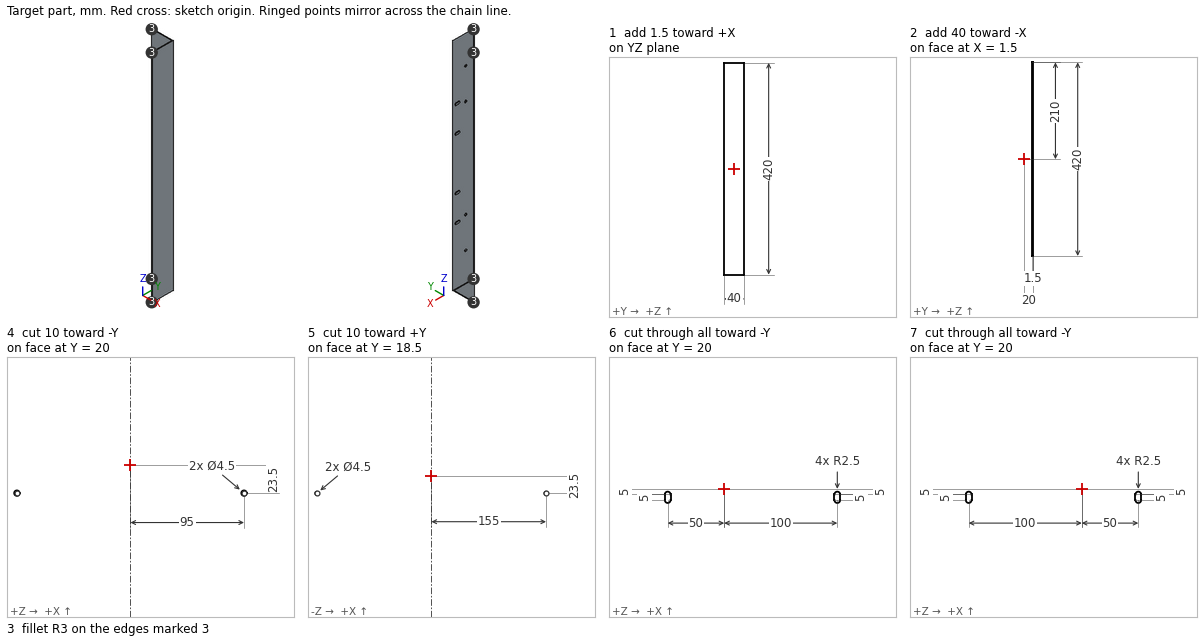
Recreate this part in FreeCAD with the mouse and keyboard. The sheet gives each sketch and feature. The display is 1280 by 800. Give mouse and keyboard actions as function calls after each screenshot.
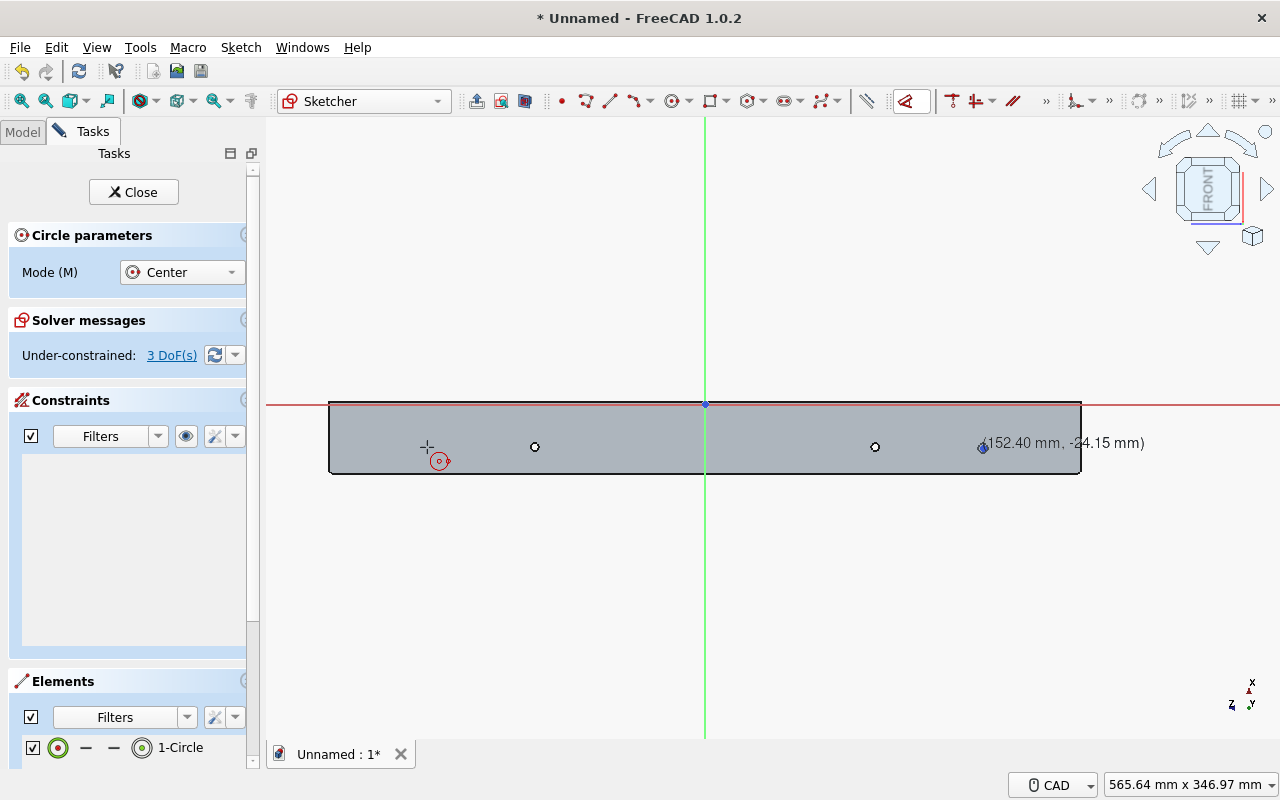
click(427, 447)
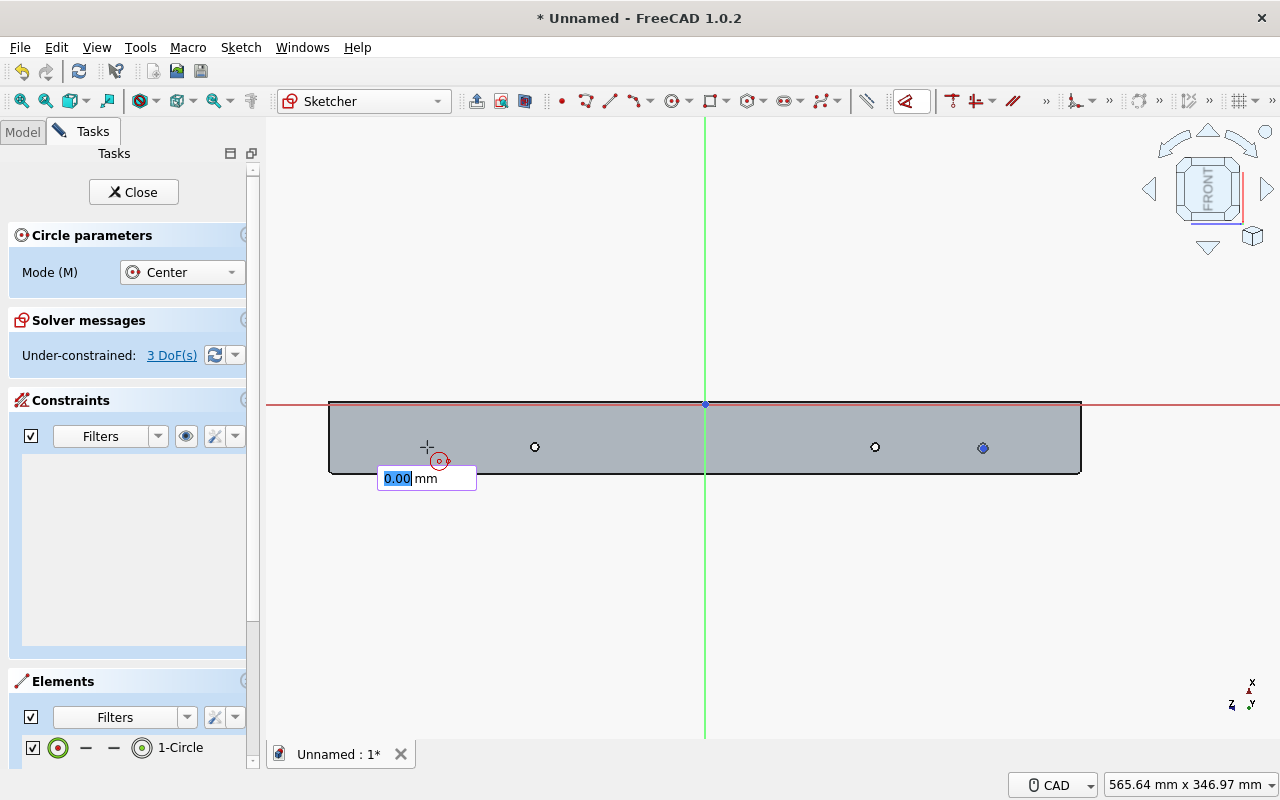
scroll(430, 444, up, 7)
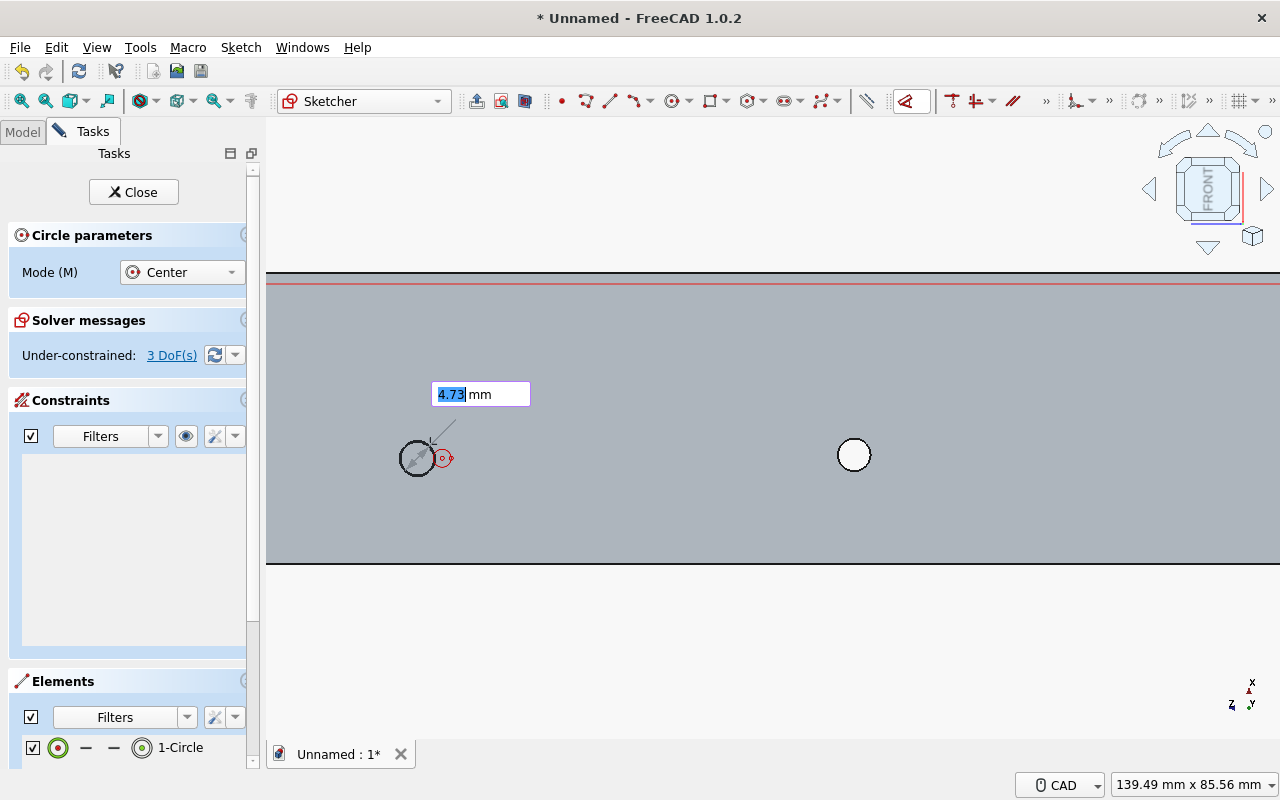
click(430, 443)
key(Escape)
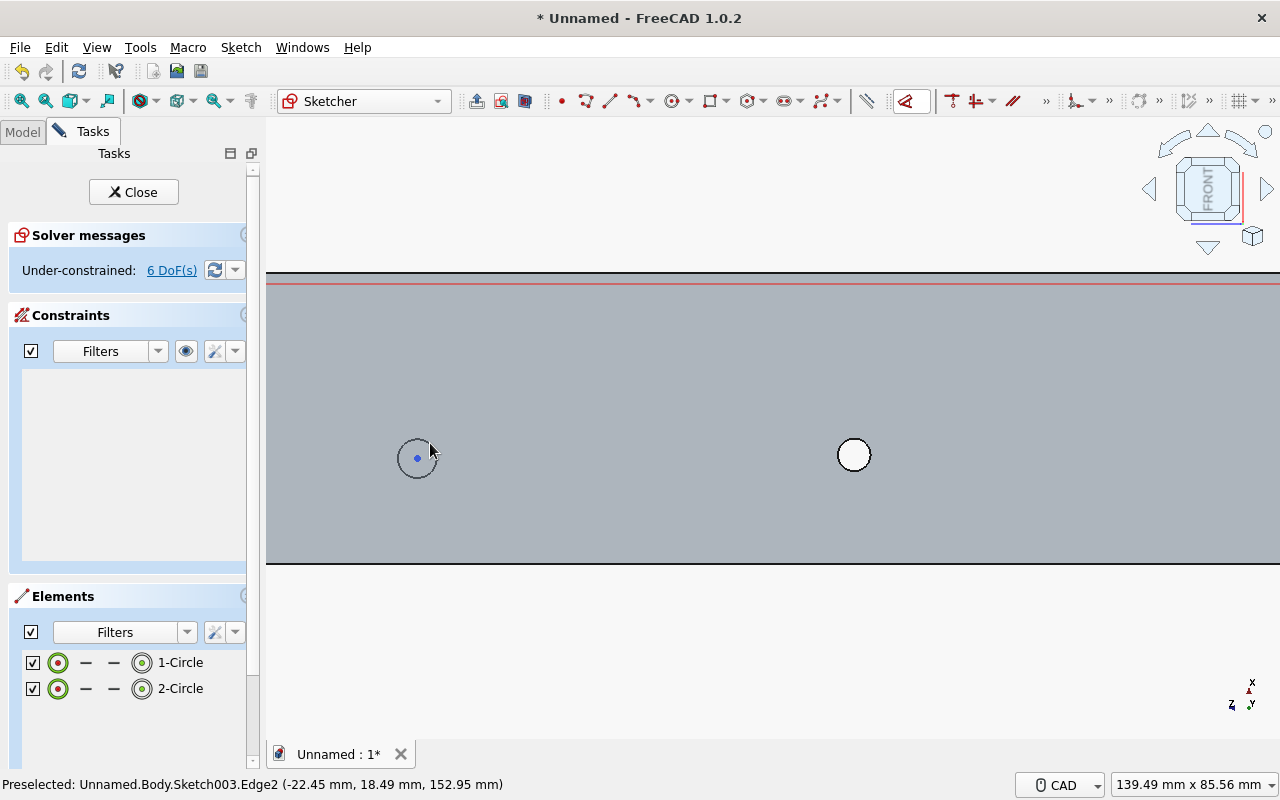
scroll(429, 444, down, 7)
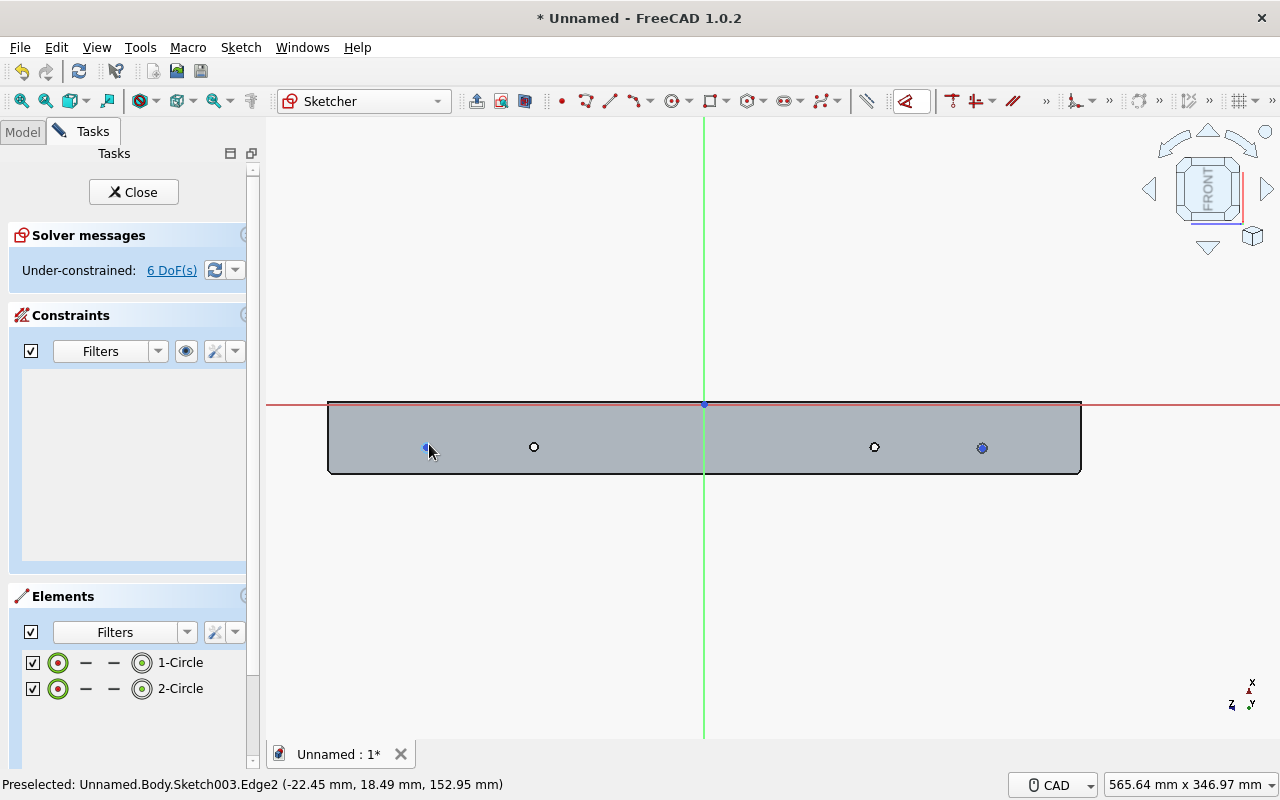
scroll(986, 445, up, 6)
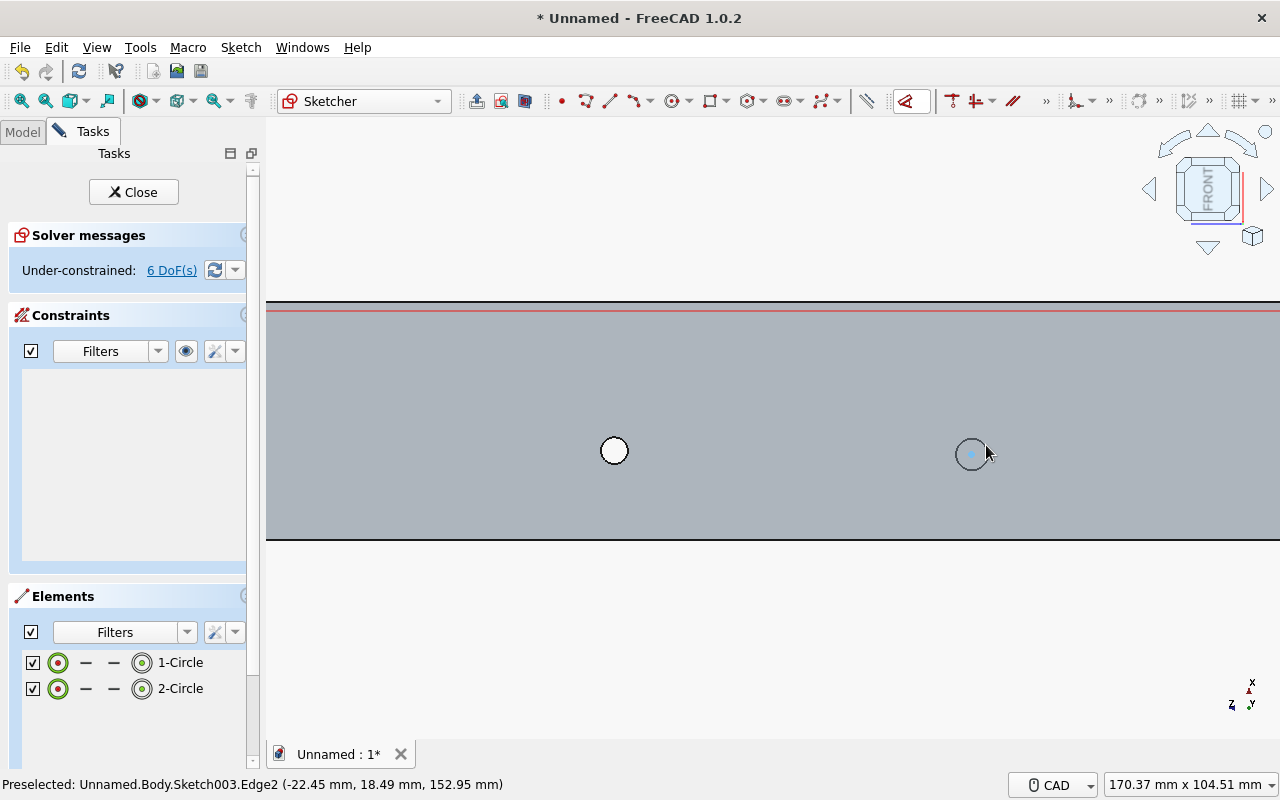
click(983, 443)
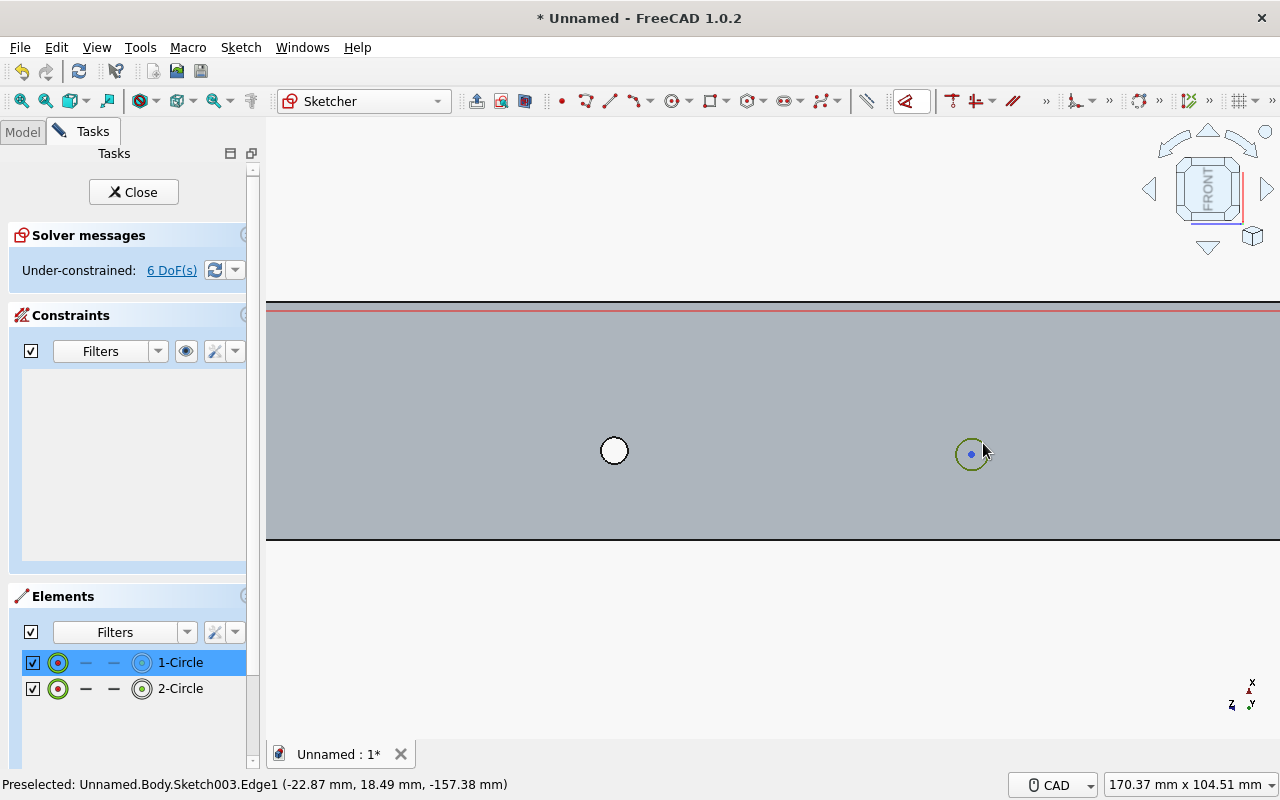
scroll(987, 445, down, 6)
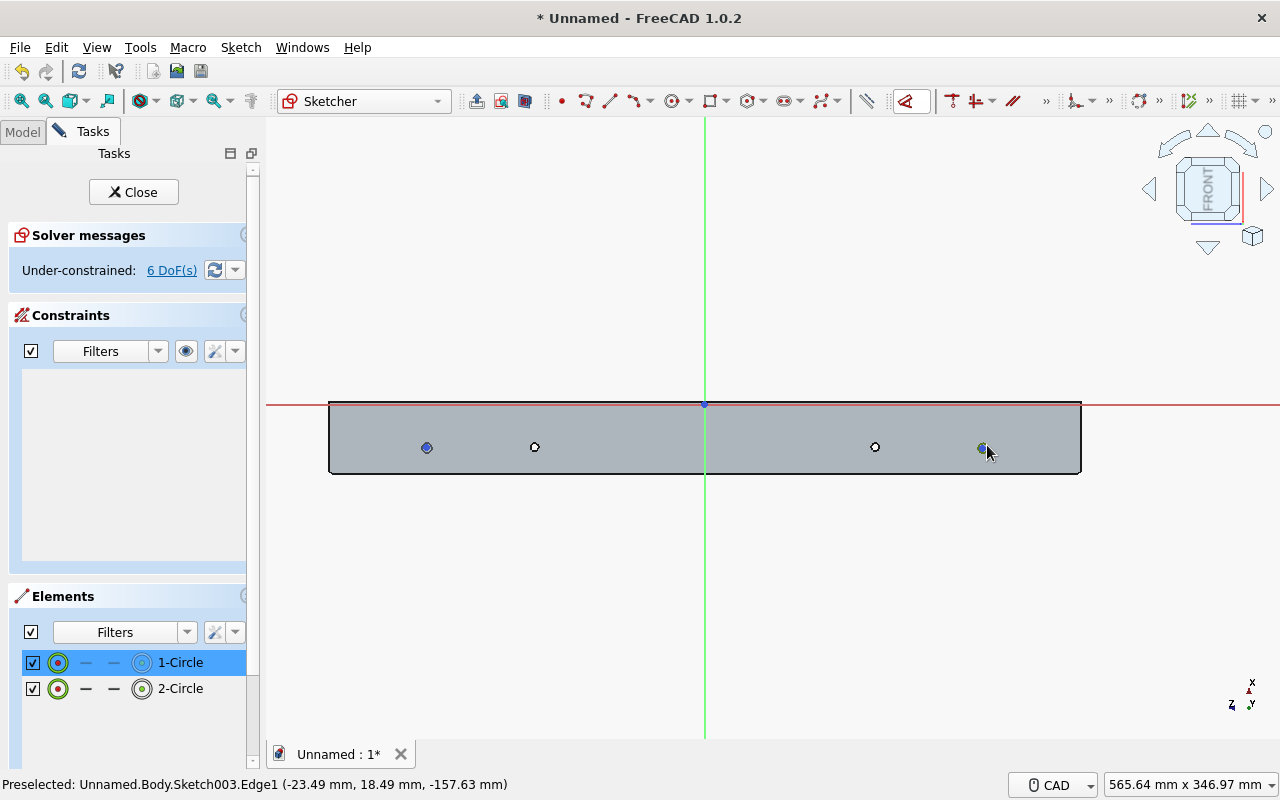
scroll(430, 445, up, 6)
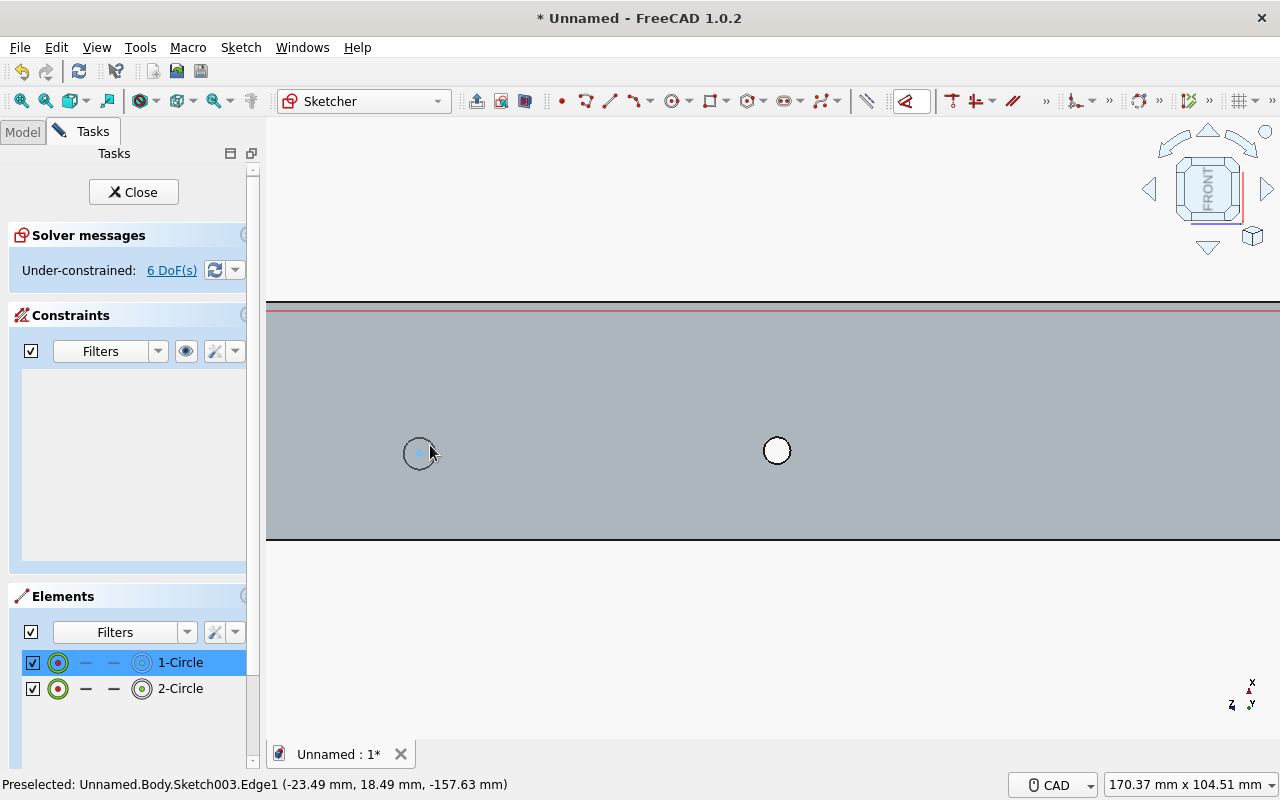
click(431, 443)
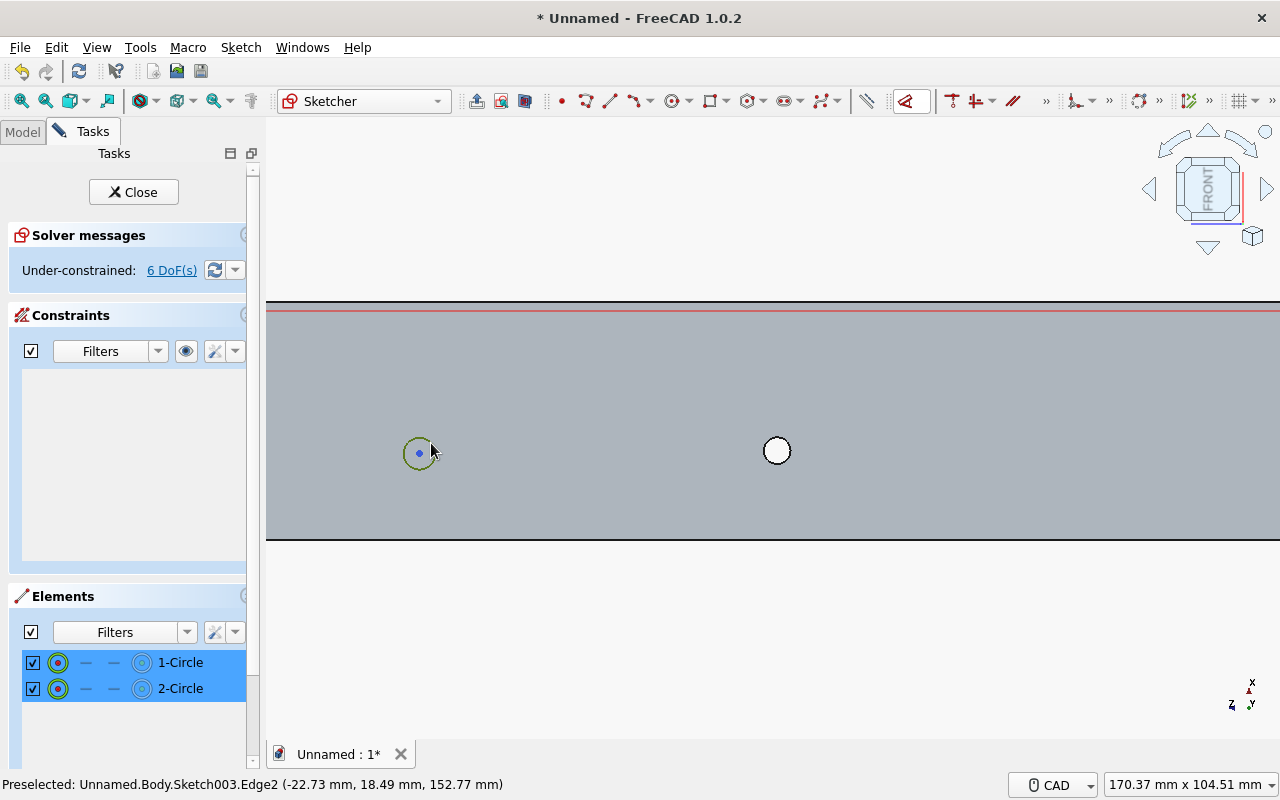
key(e)